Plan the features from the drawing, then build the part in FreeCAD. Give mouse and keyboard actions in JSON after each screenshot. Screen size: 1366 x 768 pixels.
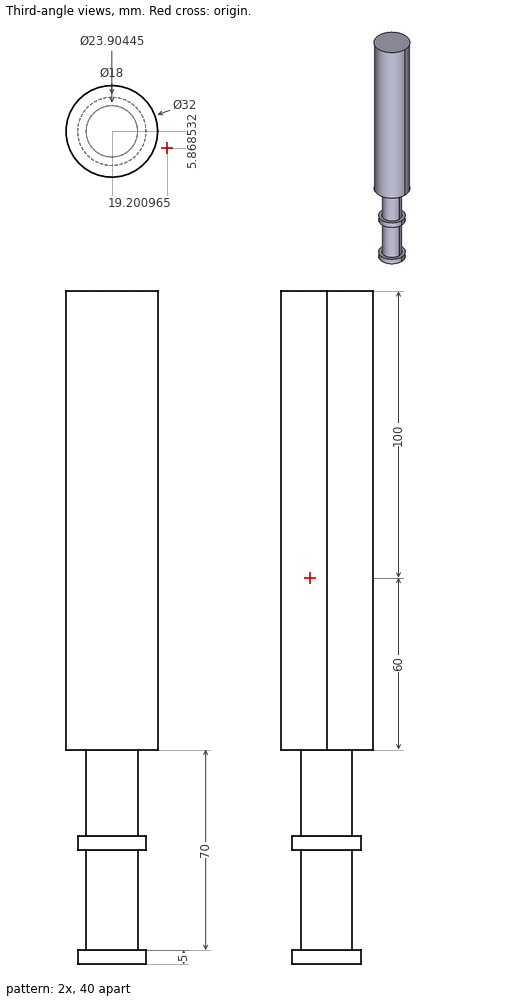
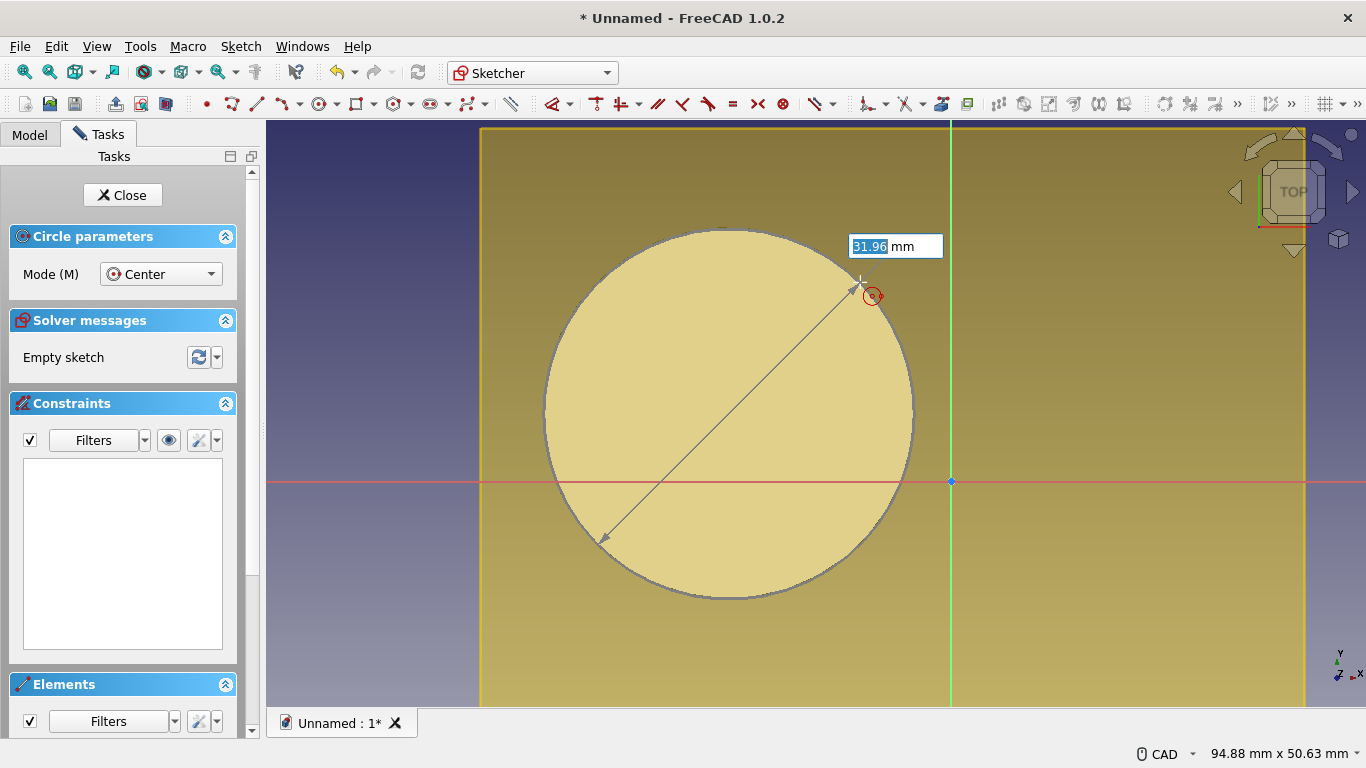
{"action": "type", "text": "32"}
{"action": "key", "text": "Return"}
{"action": "key", "text": "Escape"}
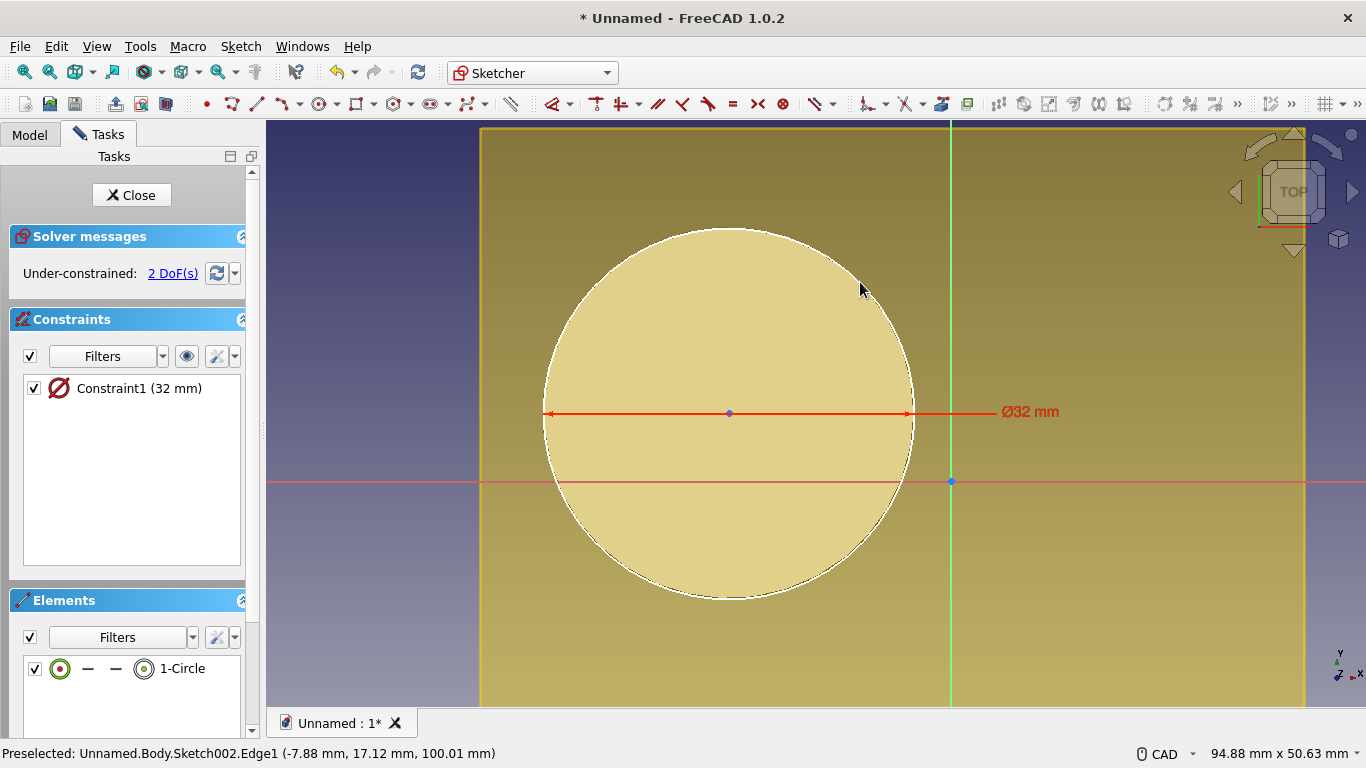
{"action": "key", "text": "d"}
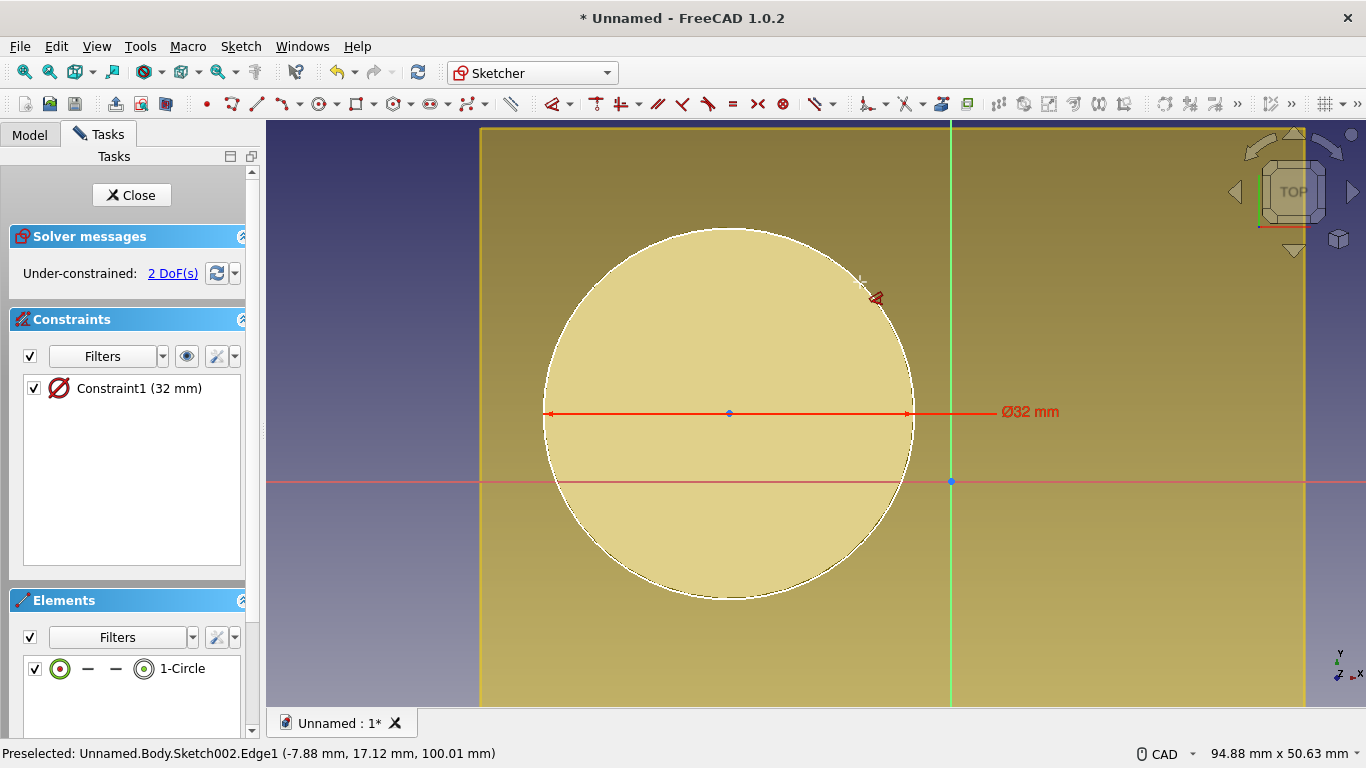
{"action": "left_click", "coordinate": [729, 414]}
{"action": "left_click", "coordinate": [985, 448]}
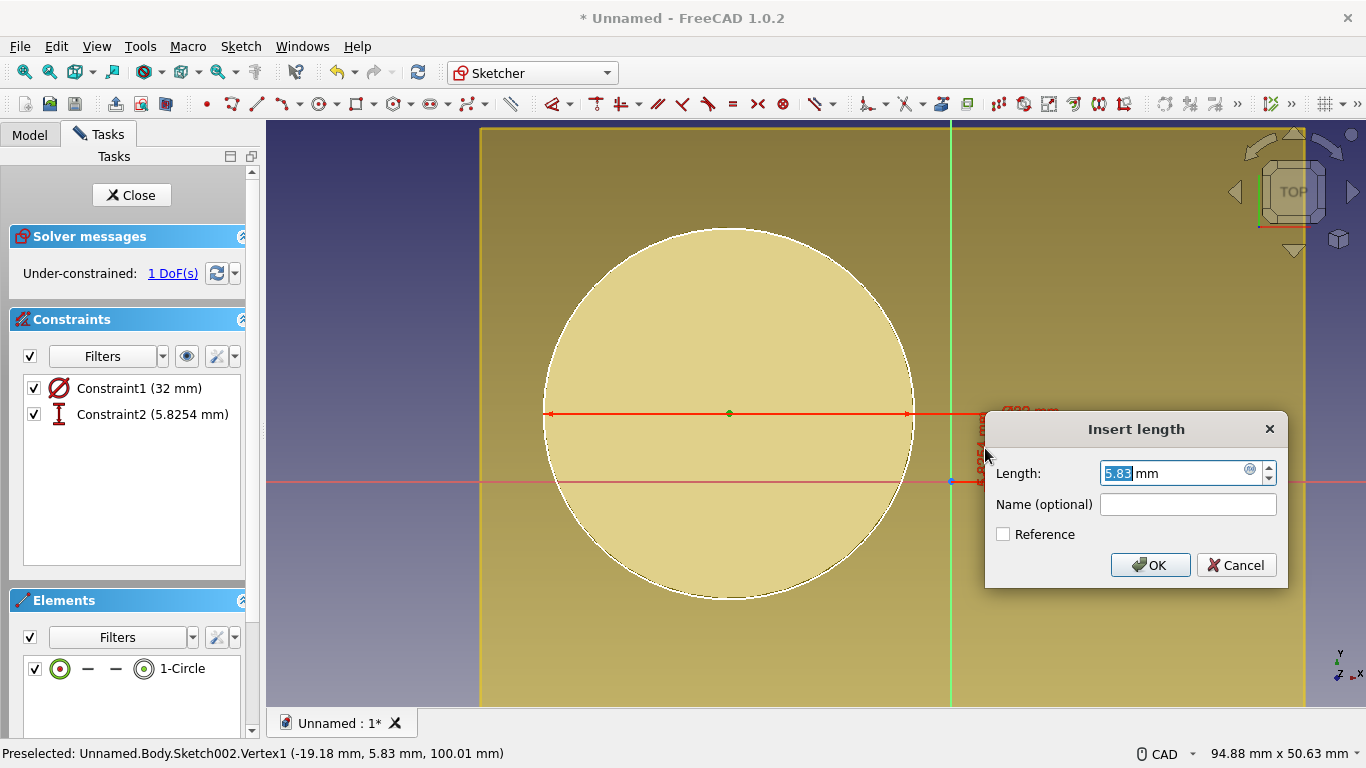
{"action": "type", "text": "5.868532"}
{"action": "key", "text": "Return"}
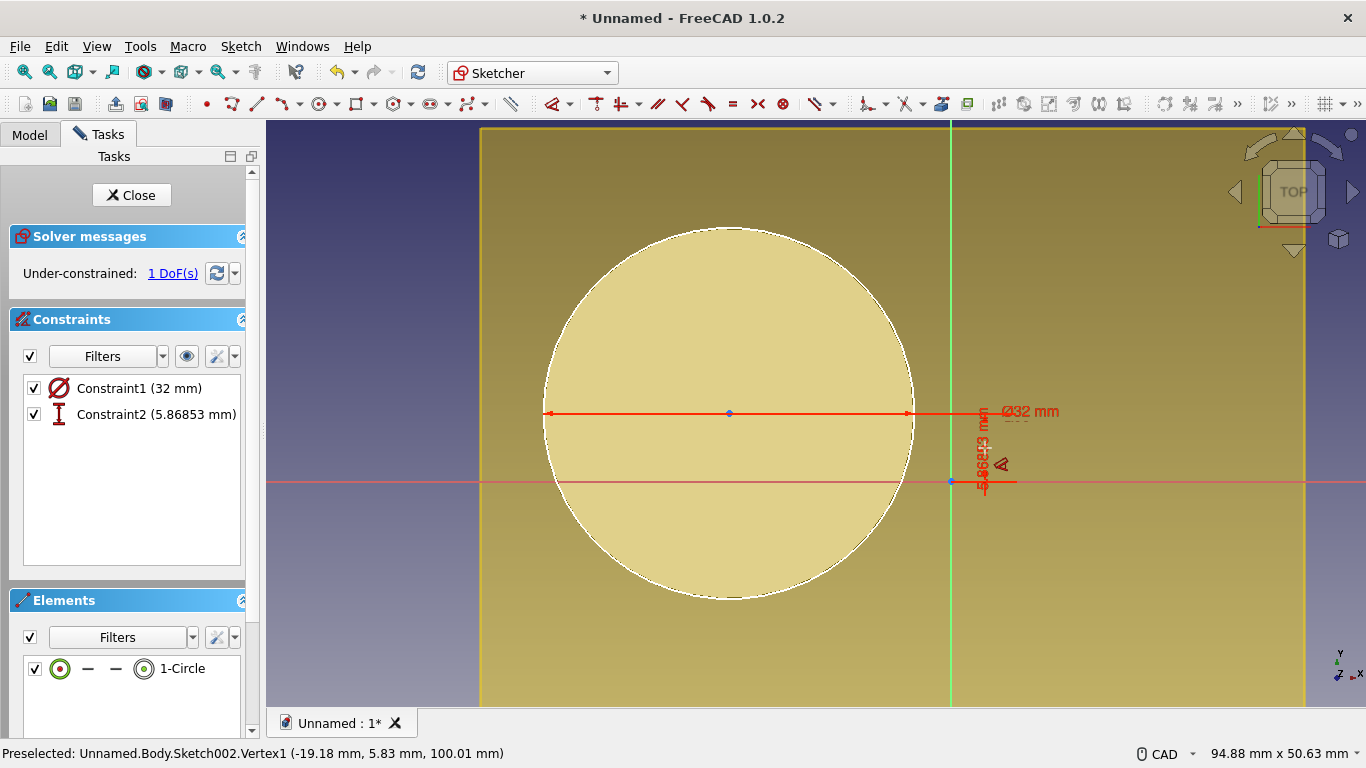
{"action": "left_click", "coordinate": [729, 413]}
{"action": "left_click", "coordinate": [840, 516]}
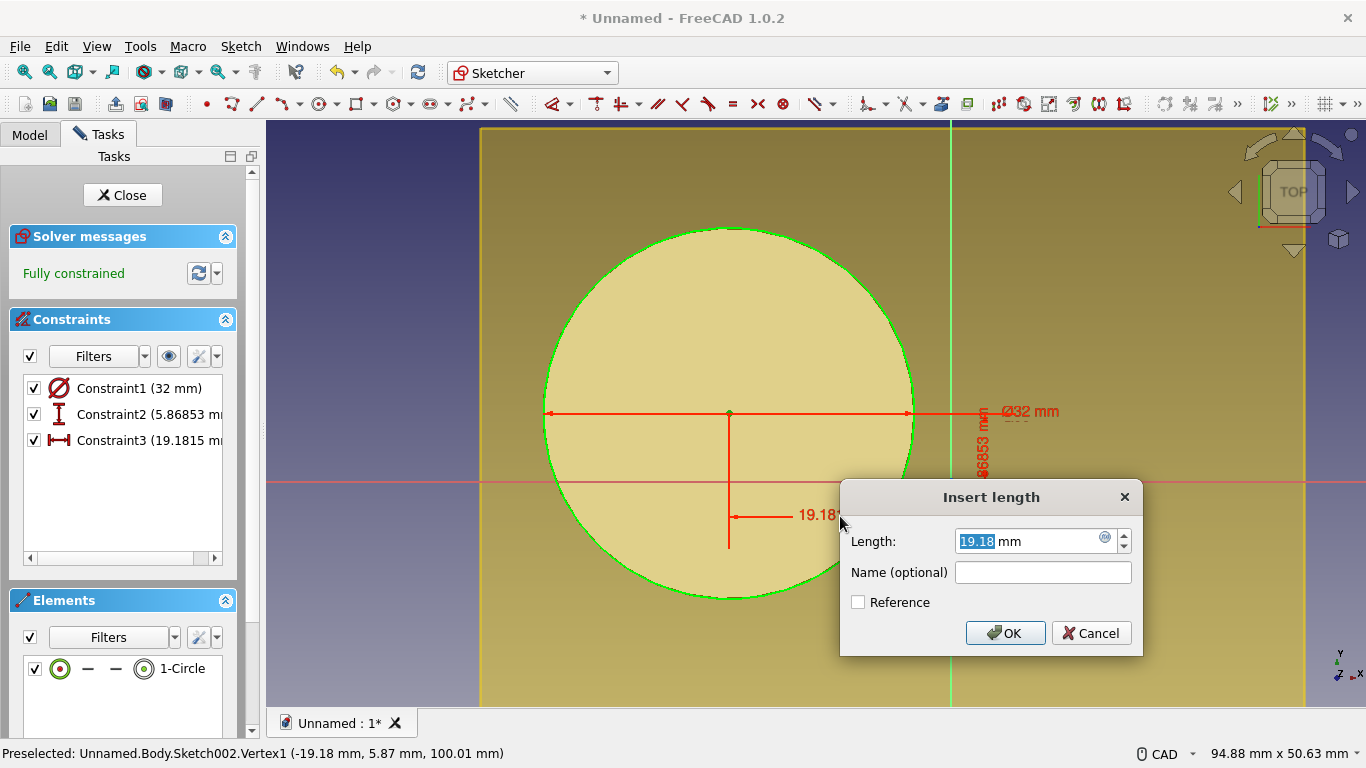
{"action": "type", "text": "19.200965"}
{"action": "key", "text": "Return"}
{"action": "key", "text": "Escape"}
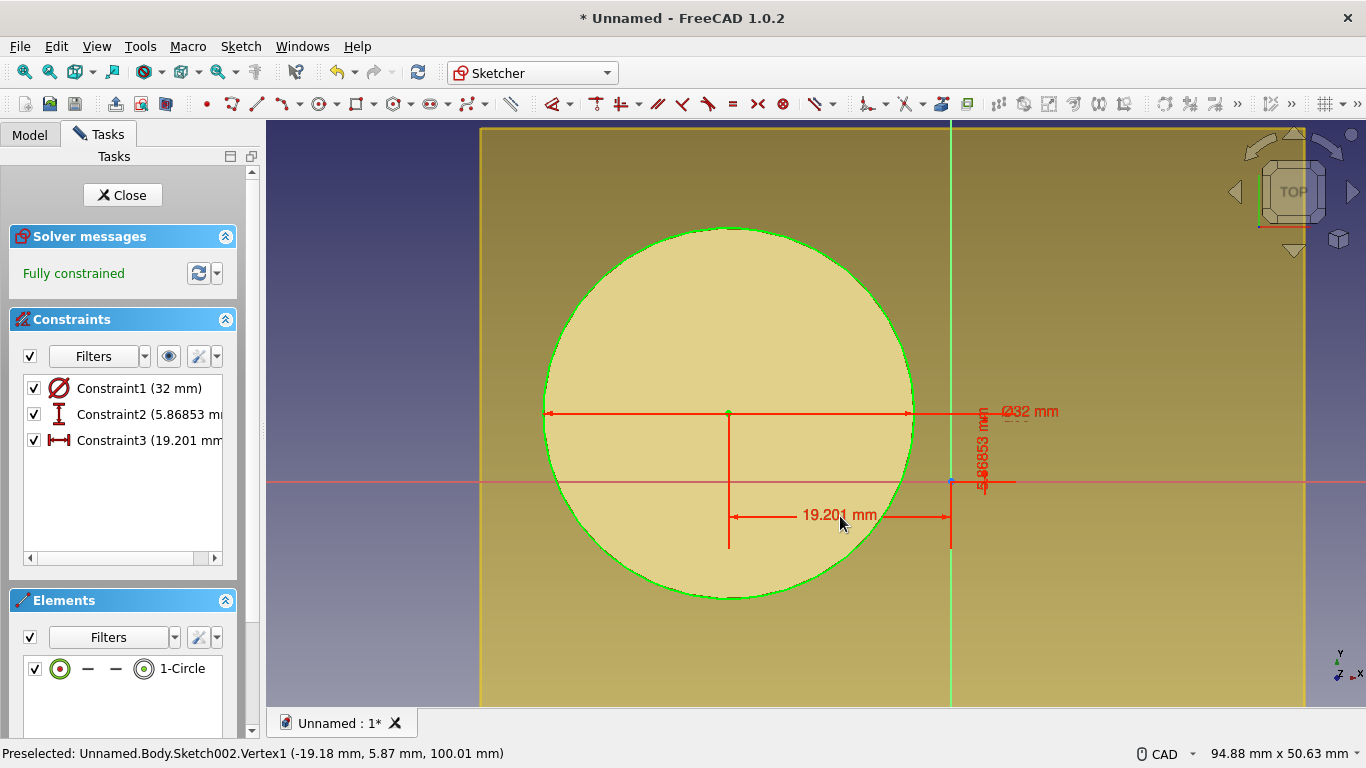
{"action": "left_click", "coordinate": [123, 195]}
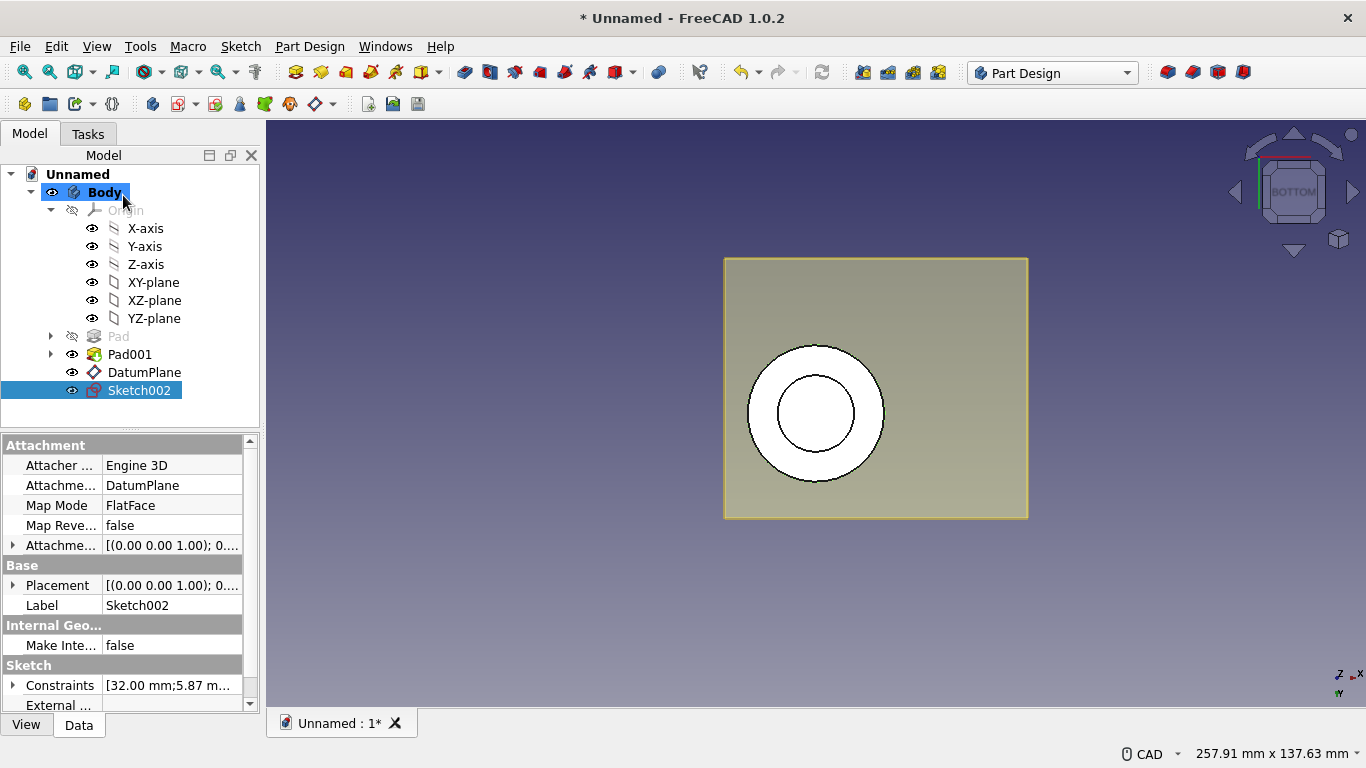
{"action": "left_click", "coordinate": [296, 72]}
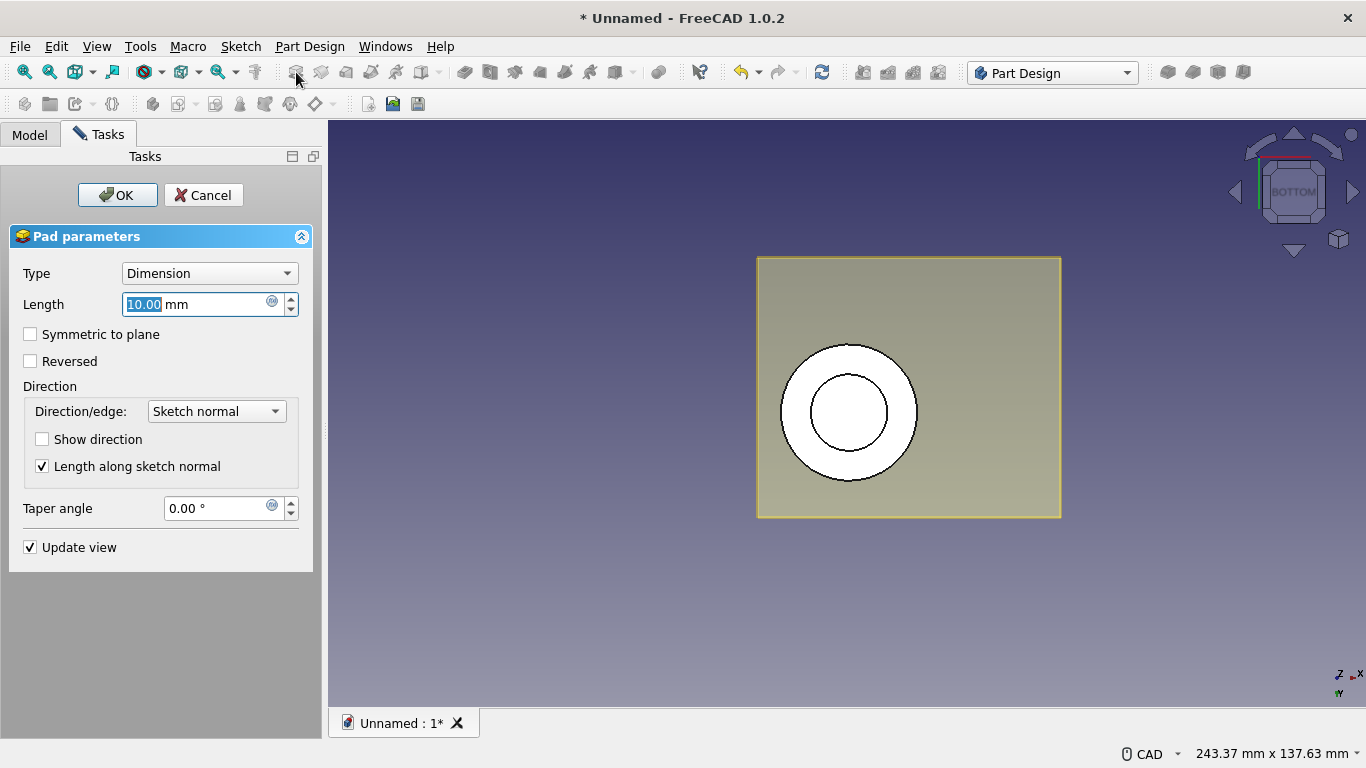
{"action": "type", "text": "100"}
{"action": "key", "text": "Tab"}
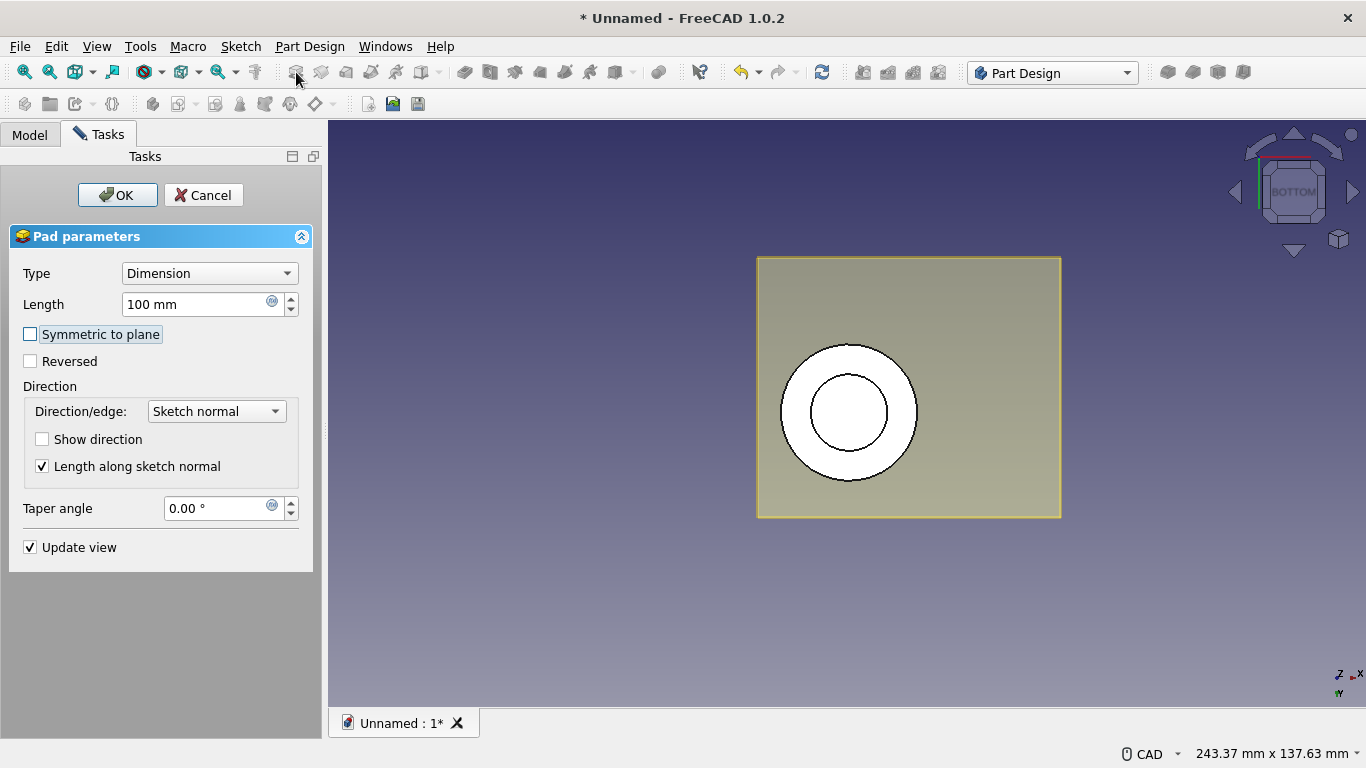
{"action": "left_click", "coordinate": [31, 361]}